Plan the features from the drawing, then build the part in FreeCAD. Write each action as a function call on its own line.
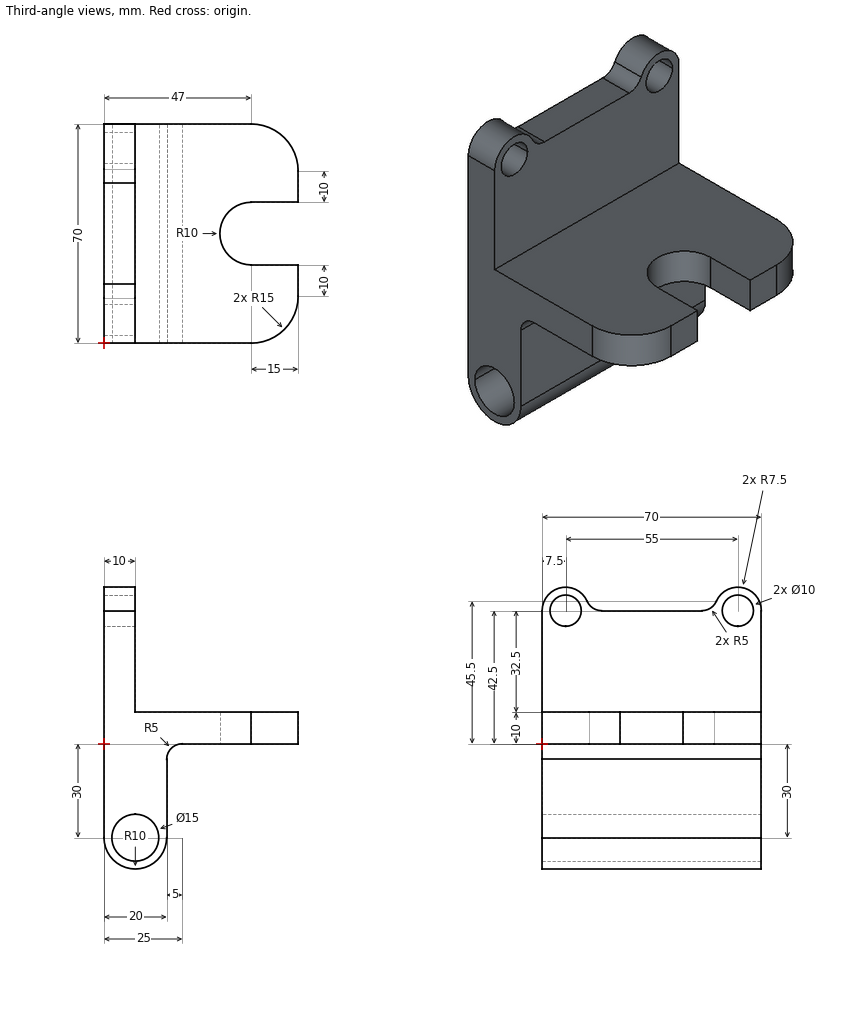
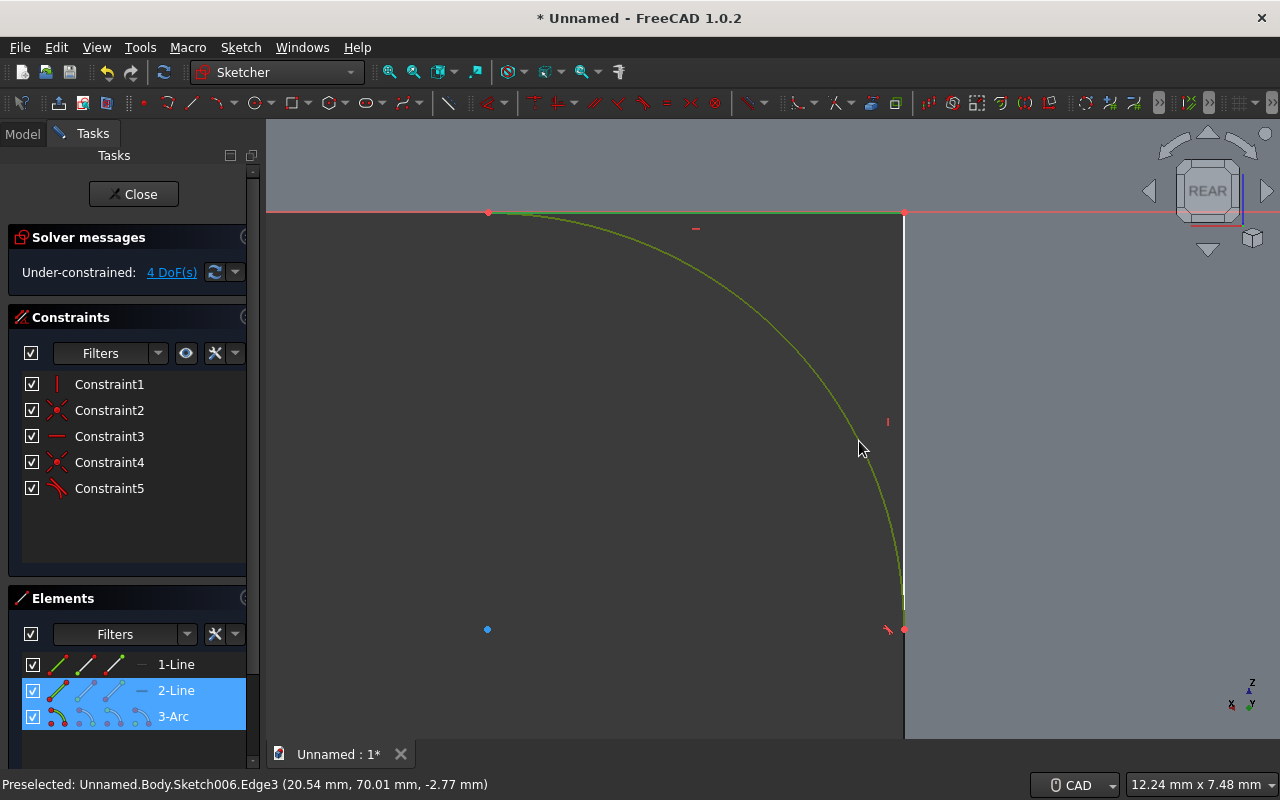
click(644, 104)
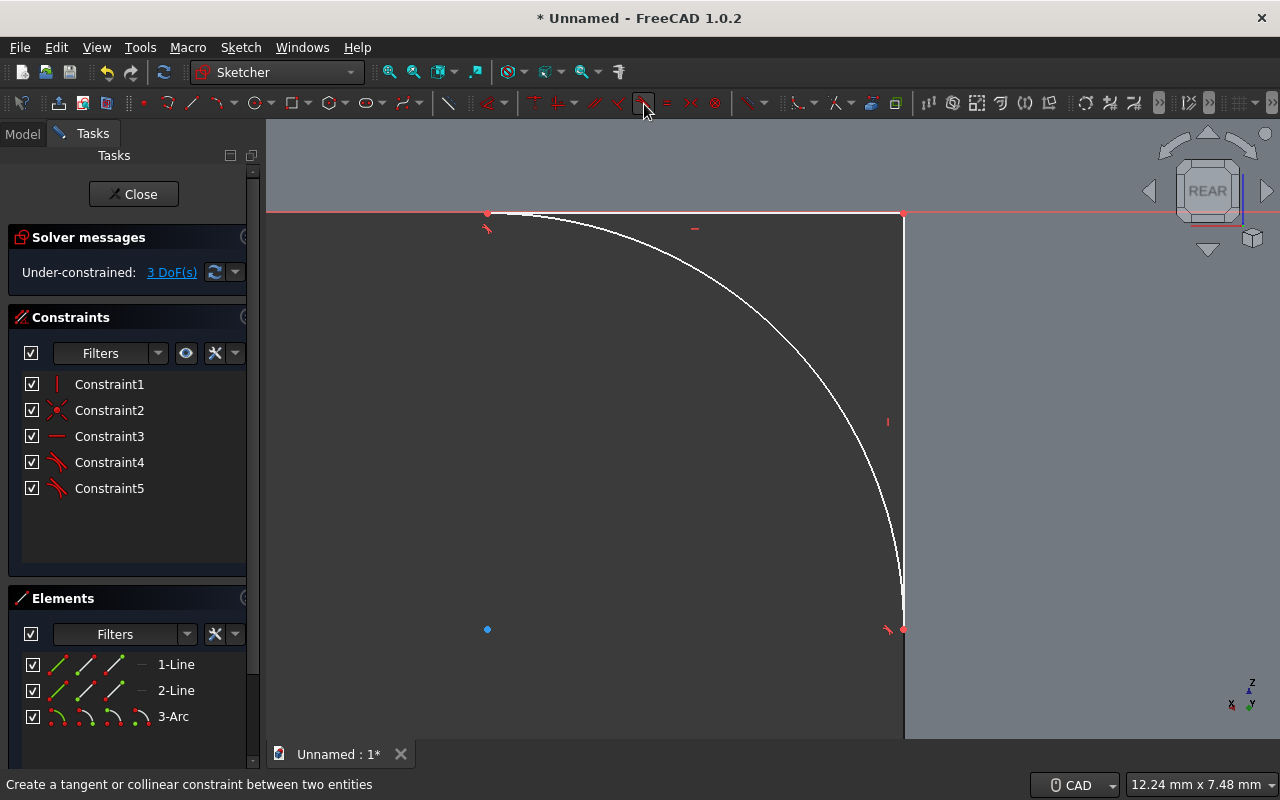
click(488, 104)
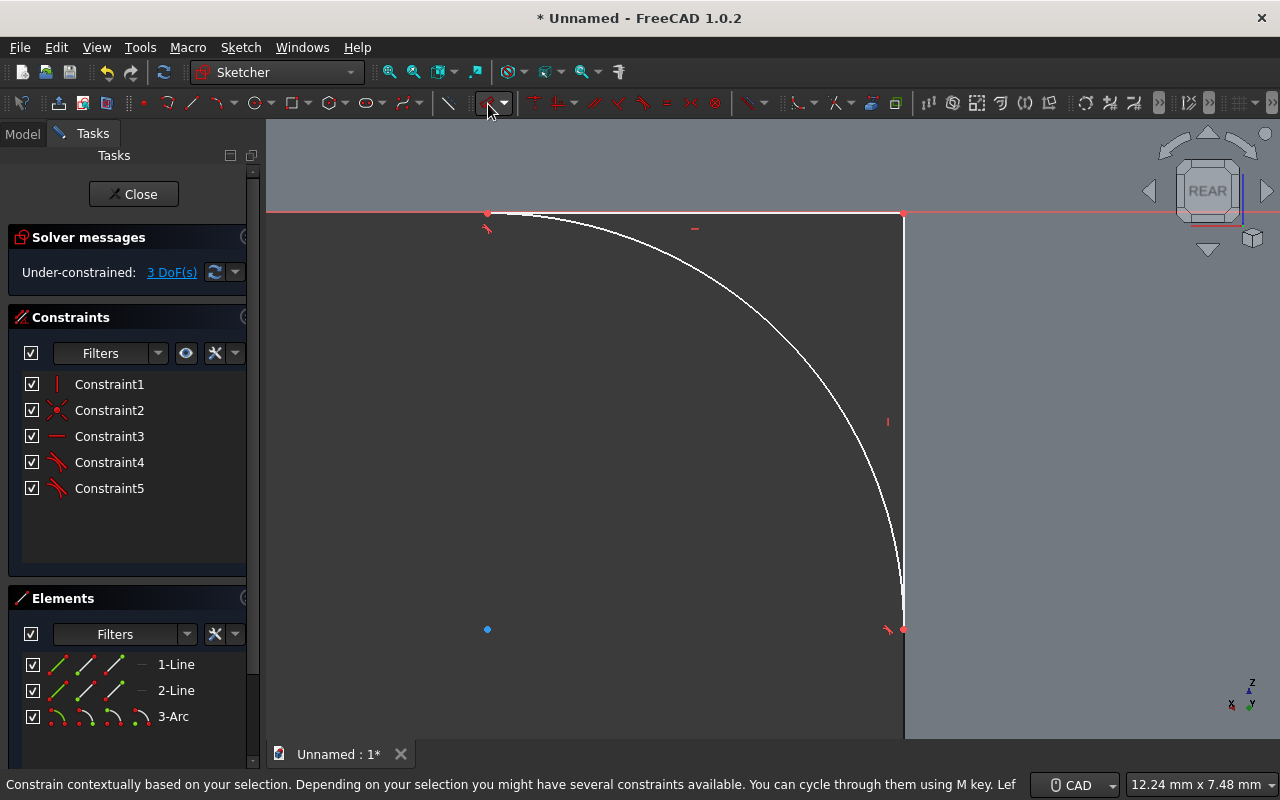
click(859, 440)
click(888, 425)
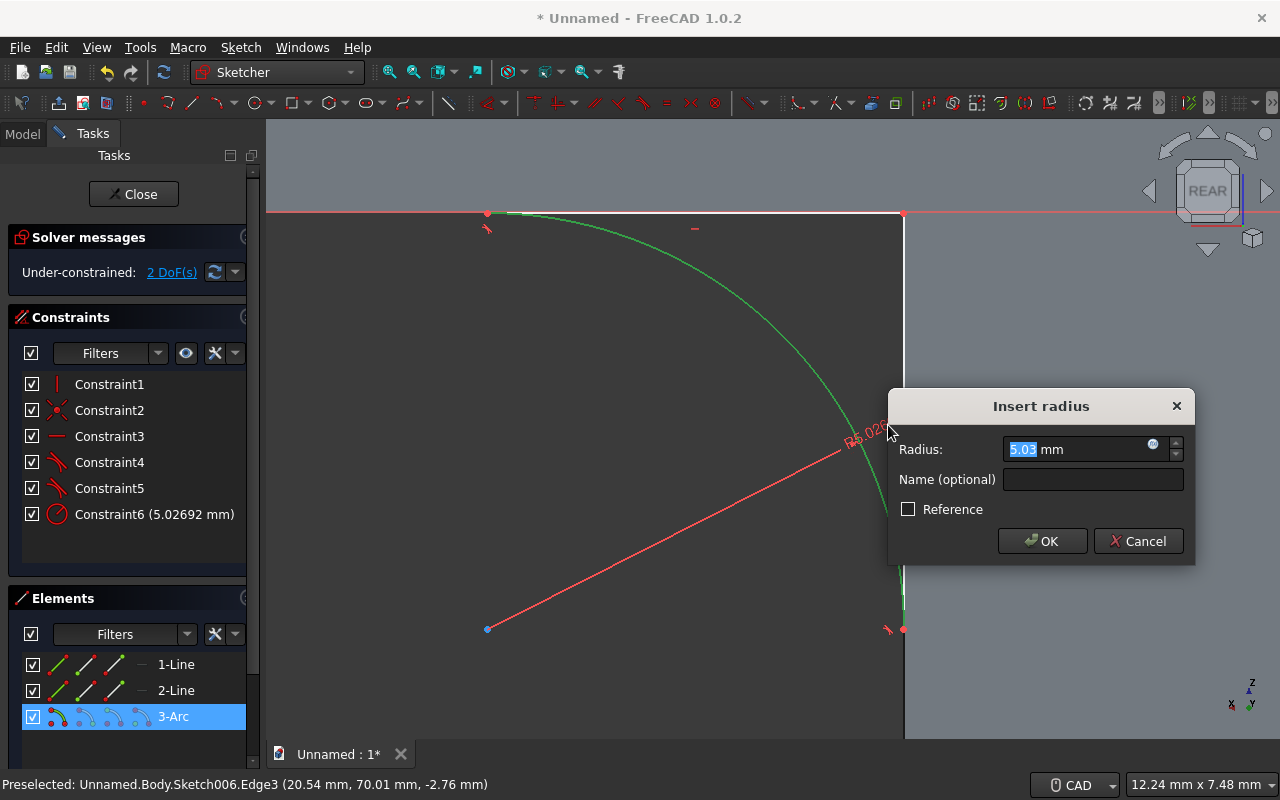
text(5)
key(Return)
key(Escape)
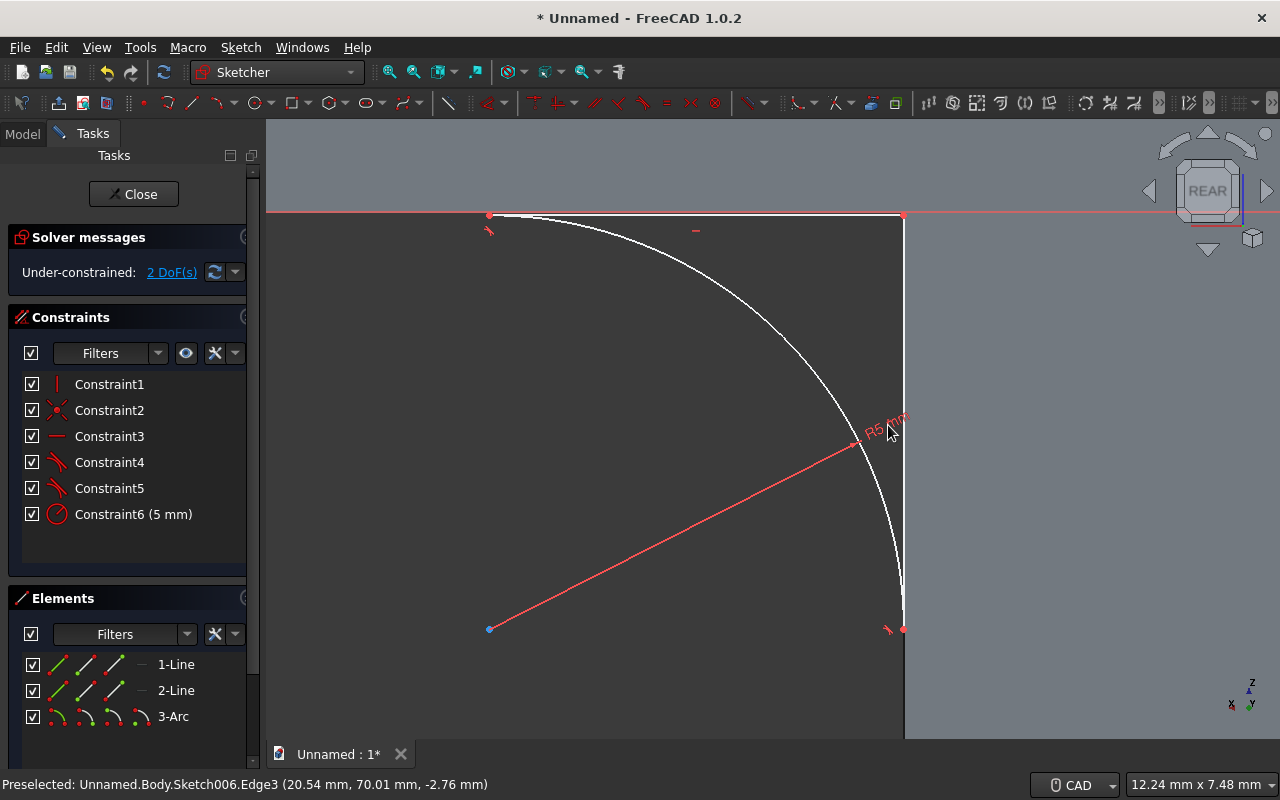
click(904, 215)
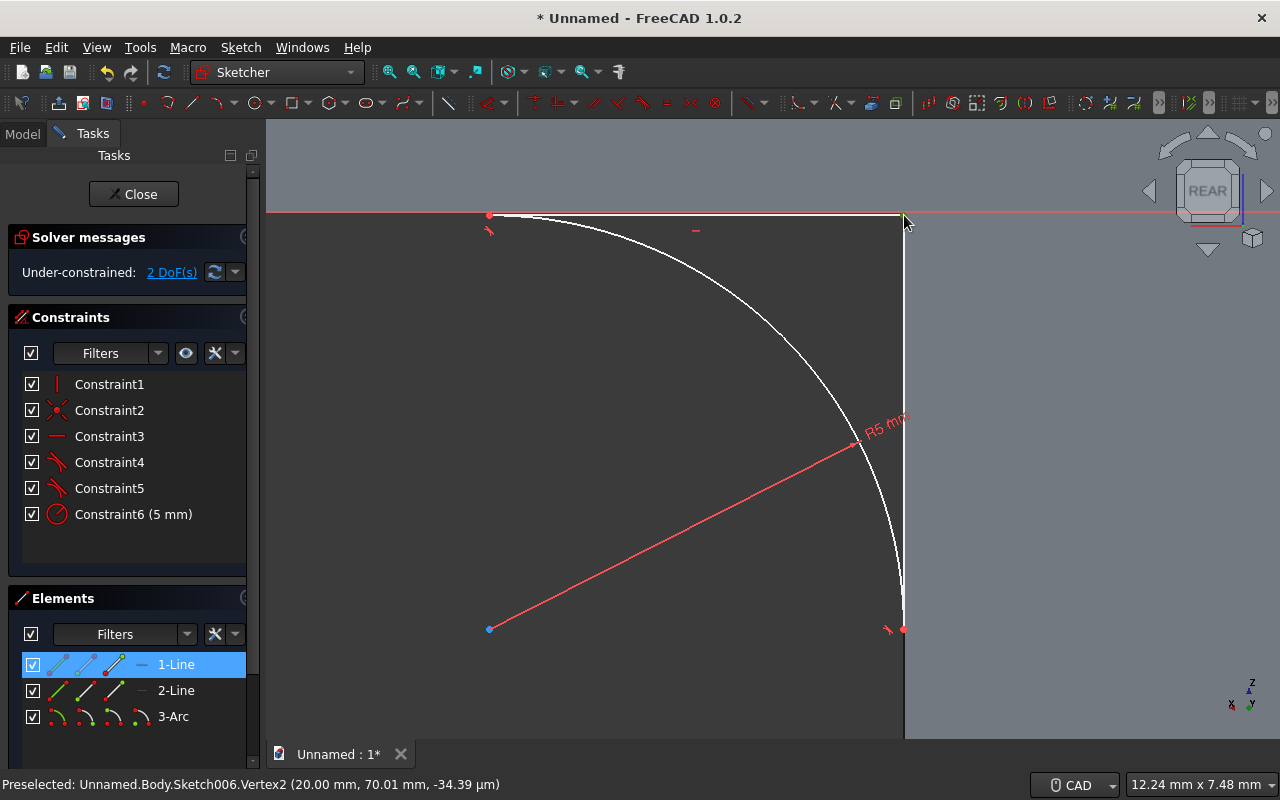
click(353, 212)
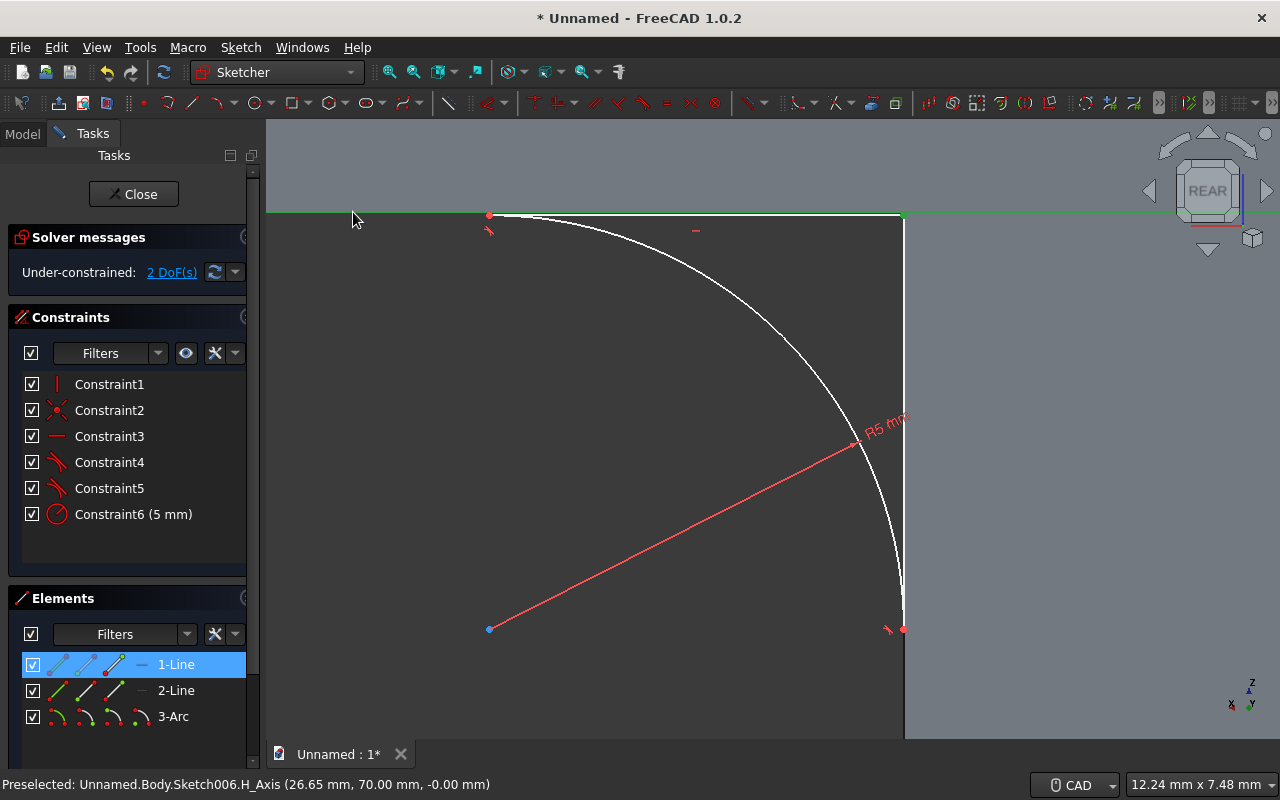
click(534, 104)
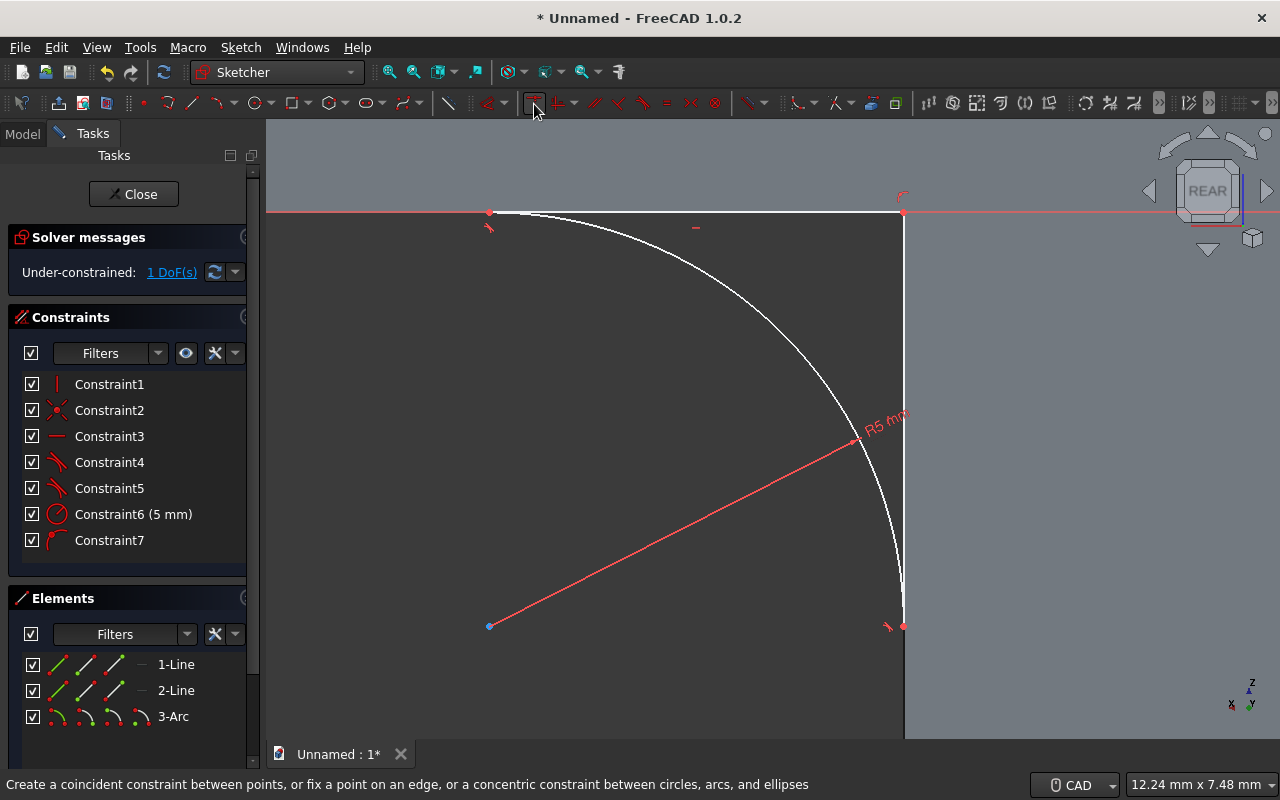
click(488, 104)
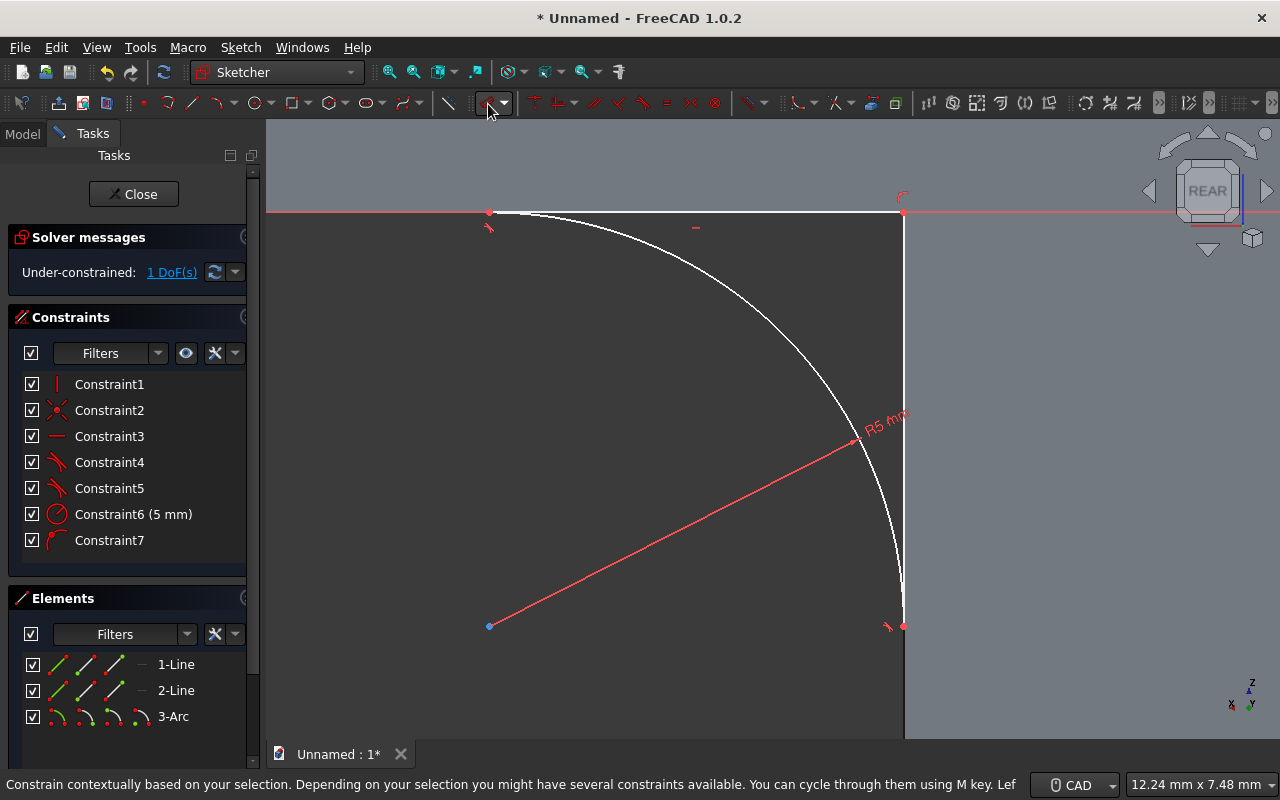
click(904, 627)
click(1009, 661)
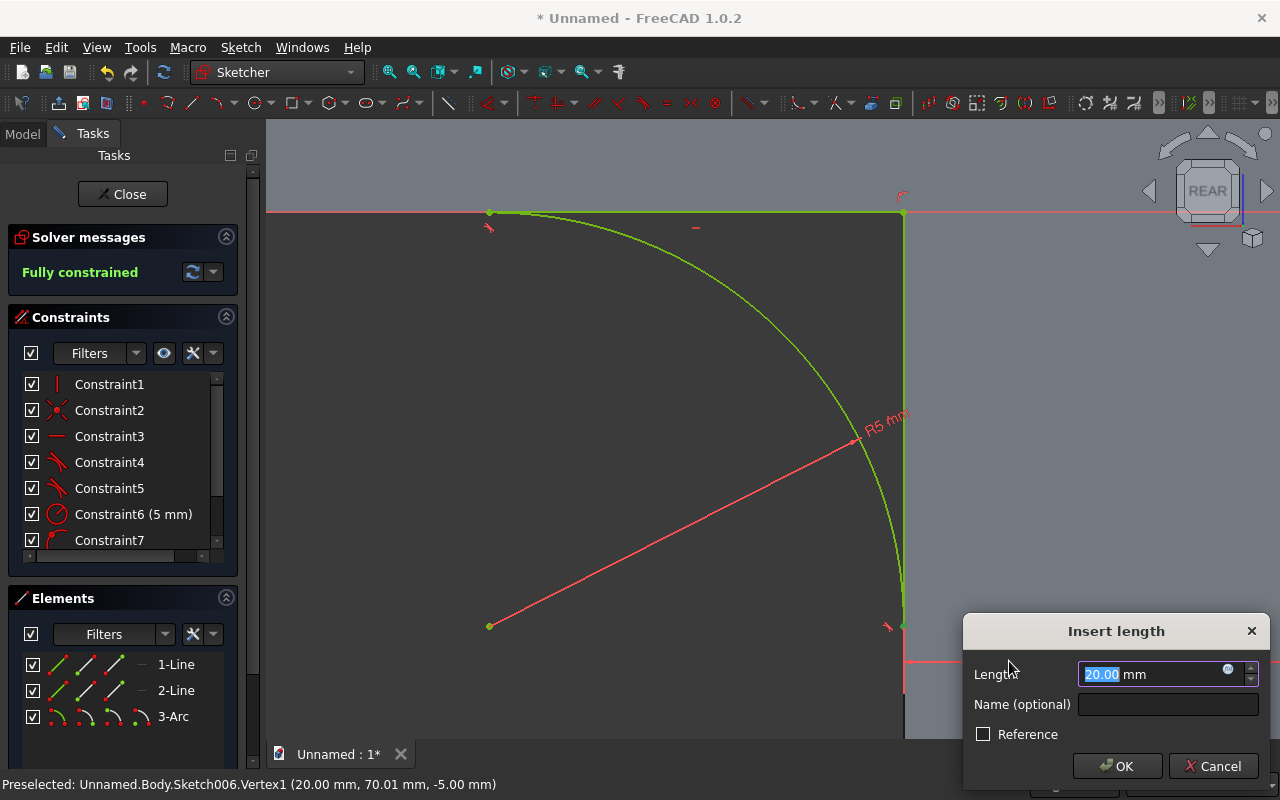
text(20)
key(Return)
key(Escape)